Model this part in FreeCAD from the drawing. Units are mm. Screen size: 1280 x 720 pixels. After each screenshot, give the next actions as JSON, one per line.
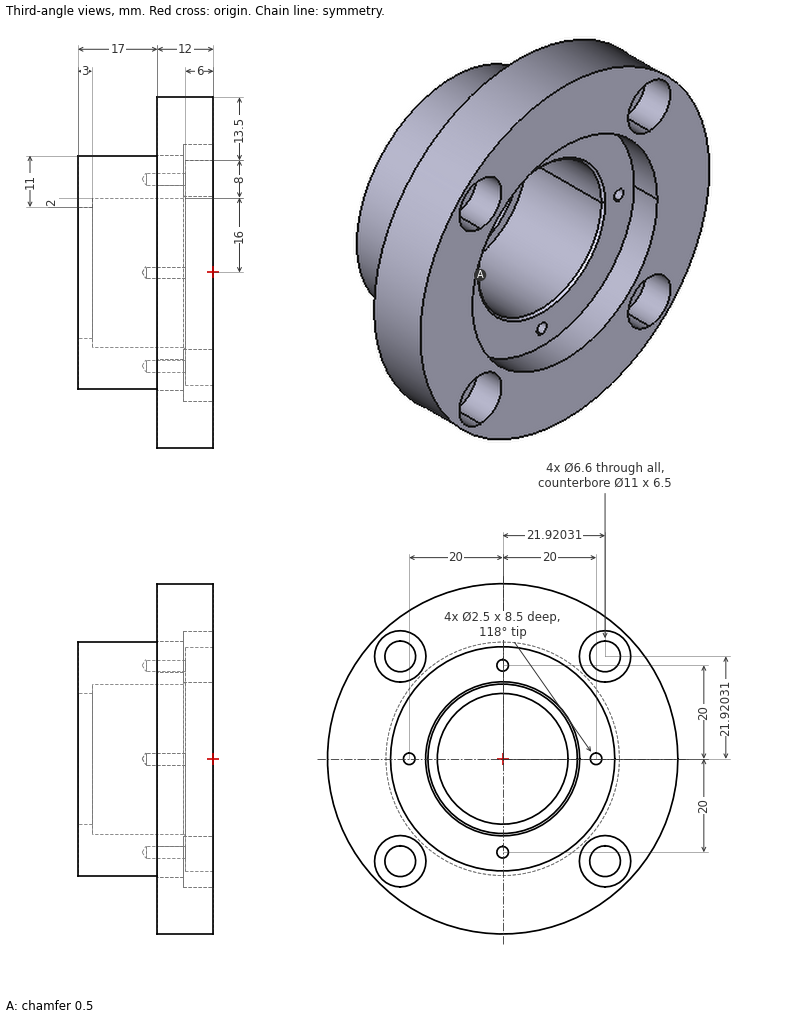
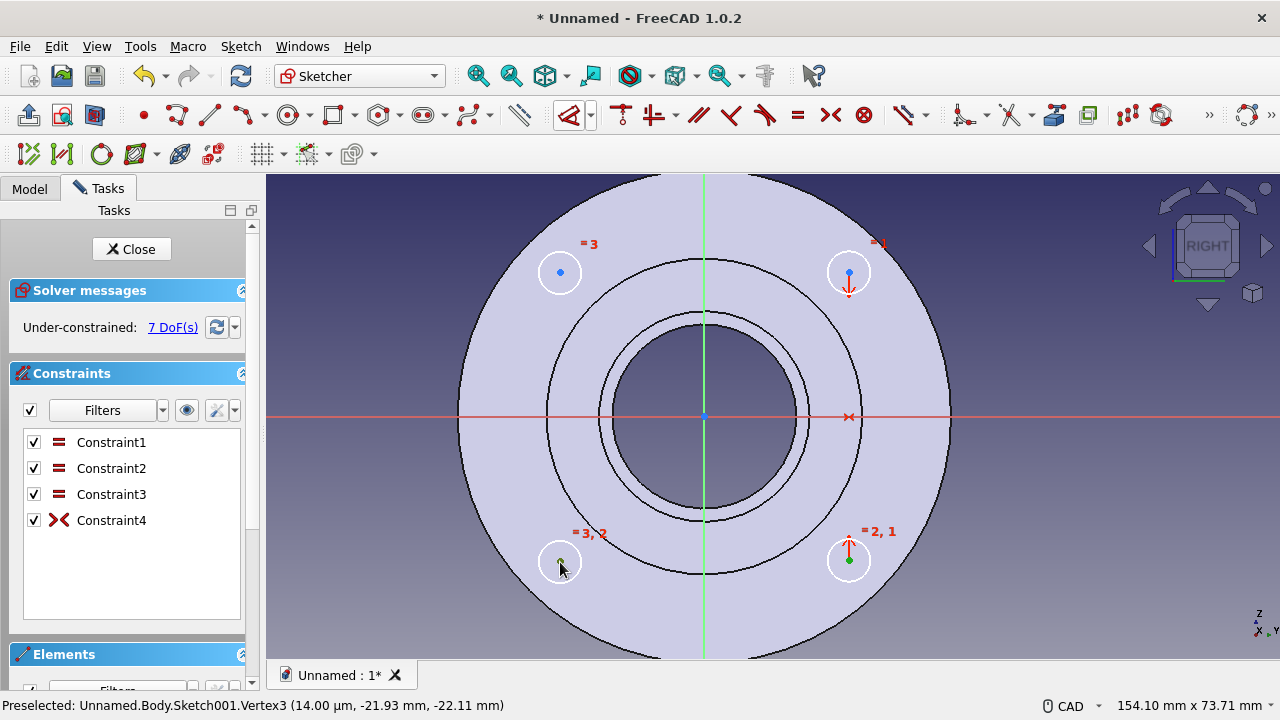
{"action": "left_click", "coordinate": [704, 600]}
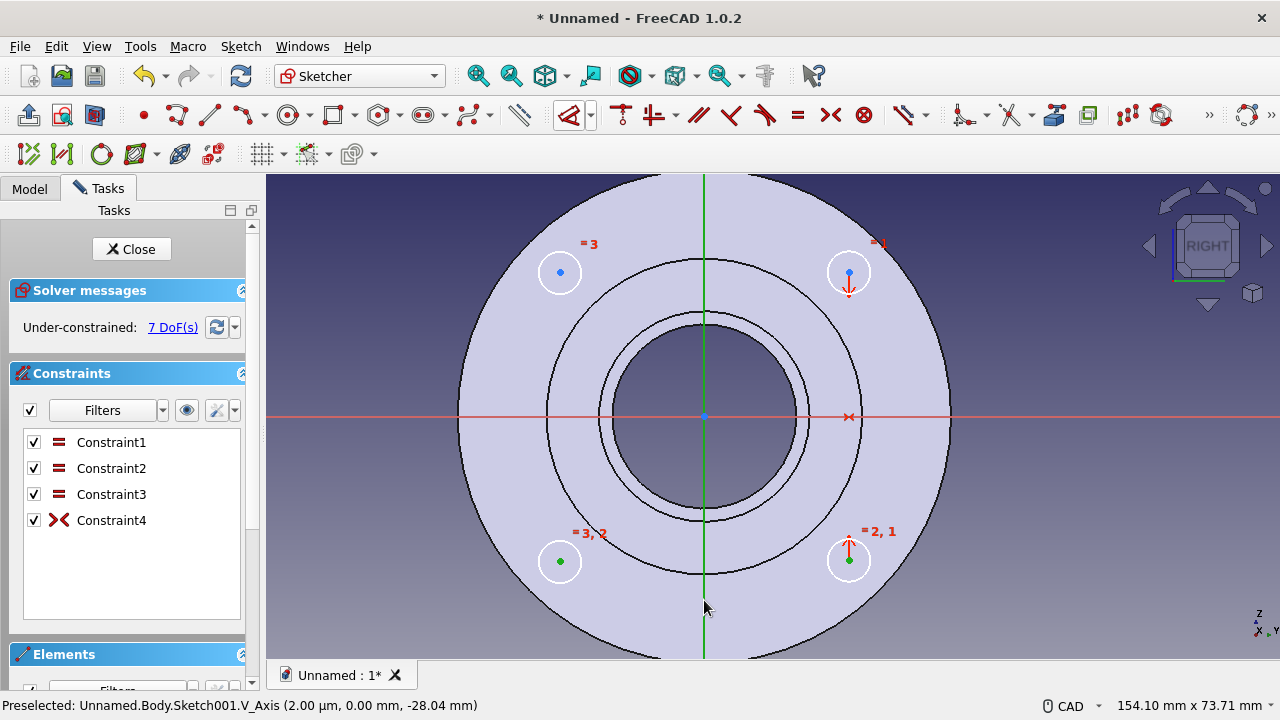
{"action": "key", "text": "s"}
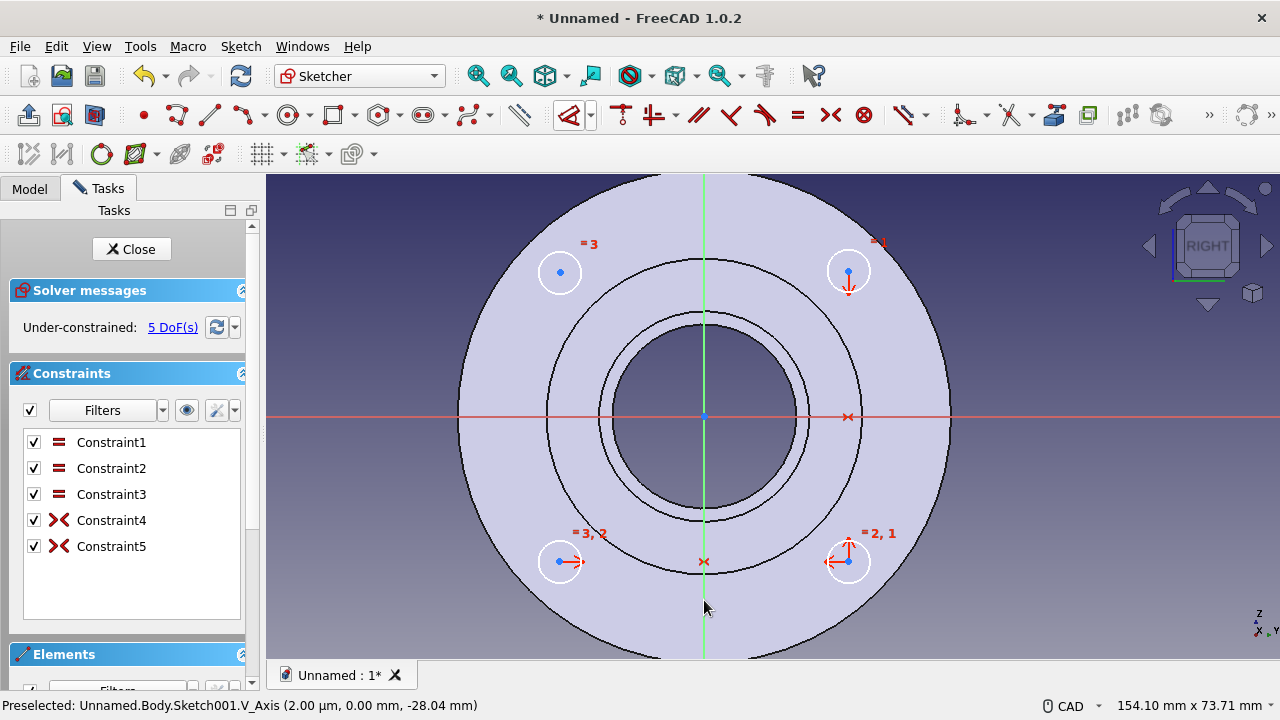
{"action": "left_click", "coordinate": [849, 271]}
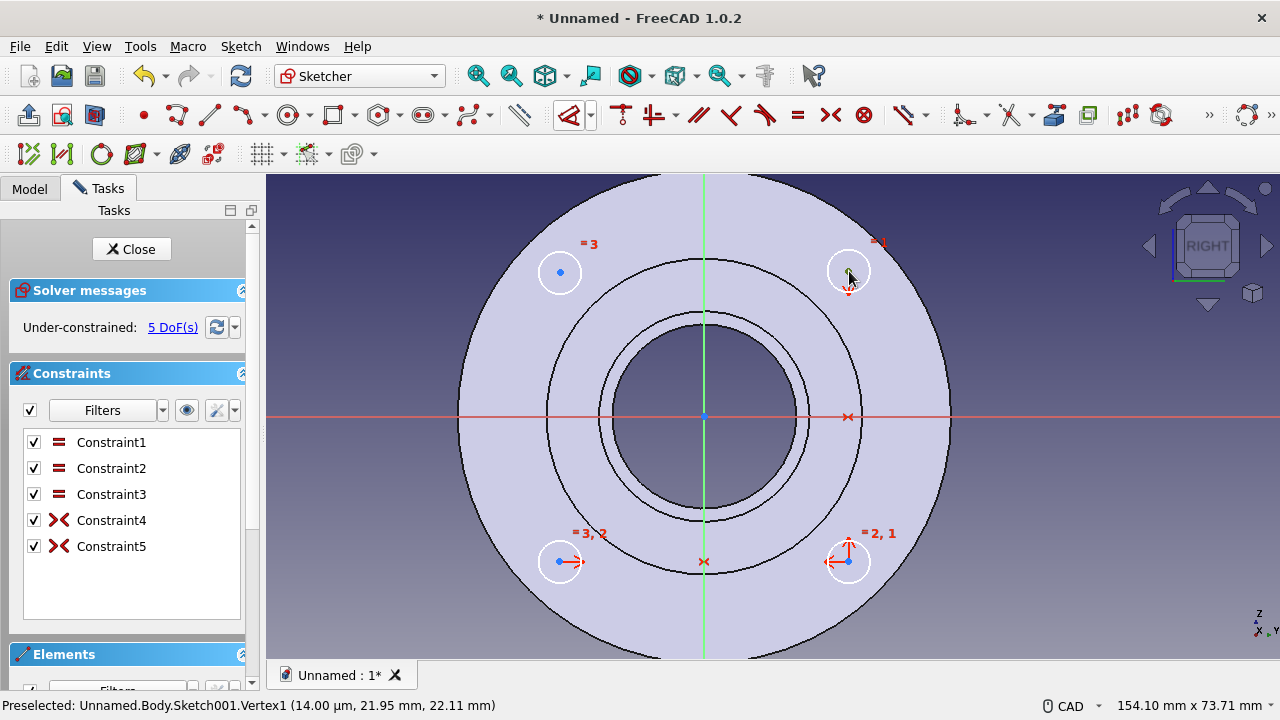
{"action": "left_click", "coordinate": [560, 273]}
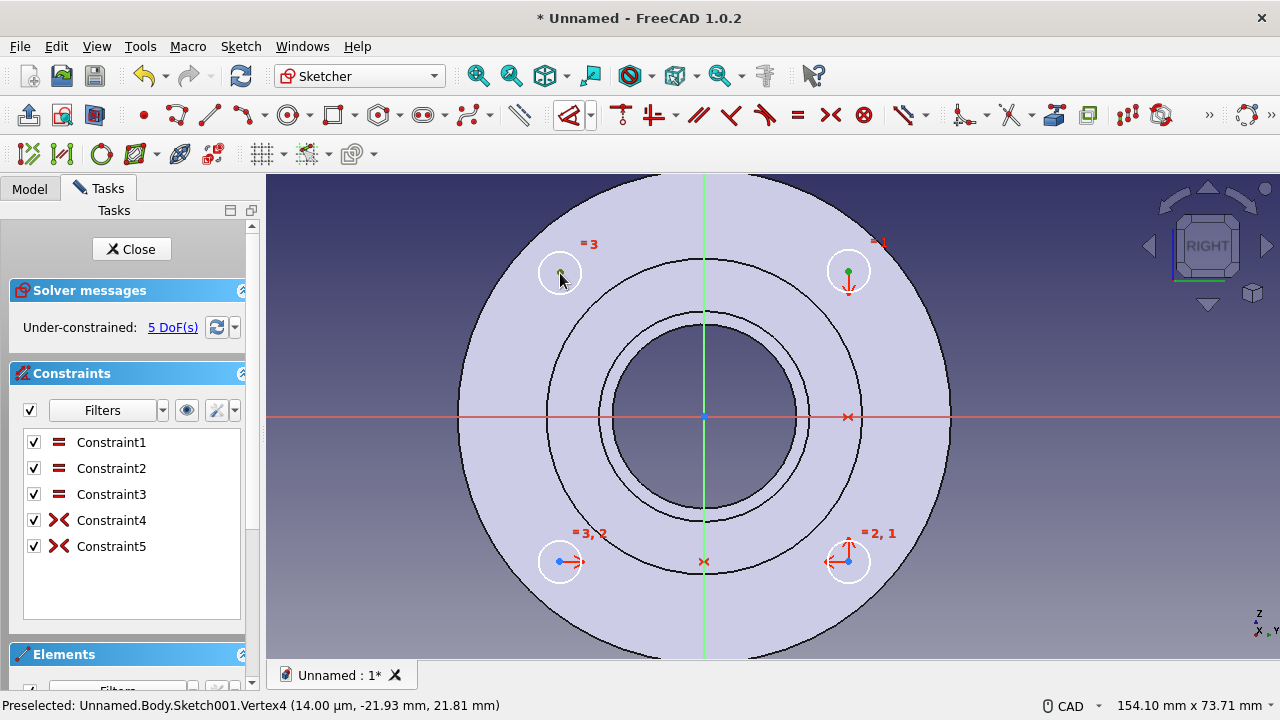
{"action": "left_click", "coordinate": [704, 600]}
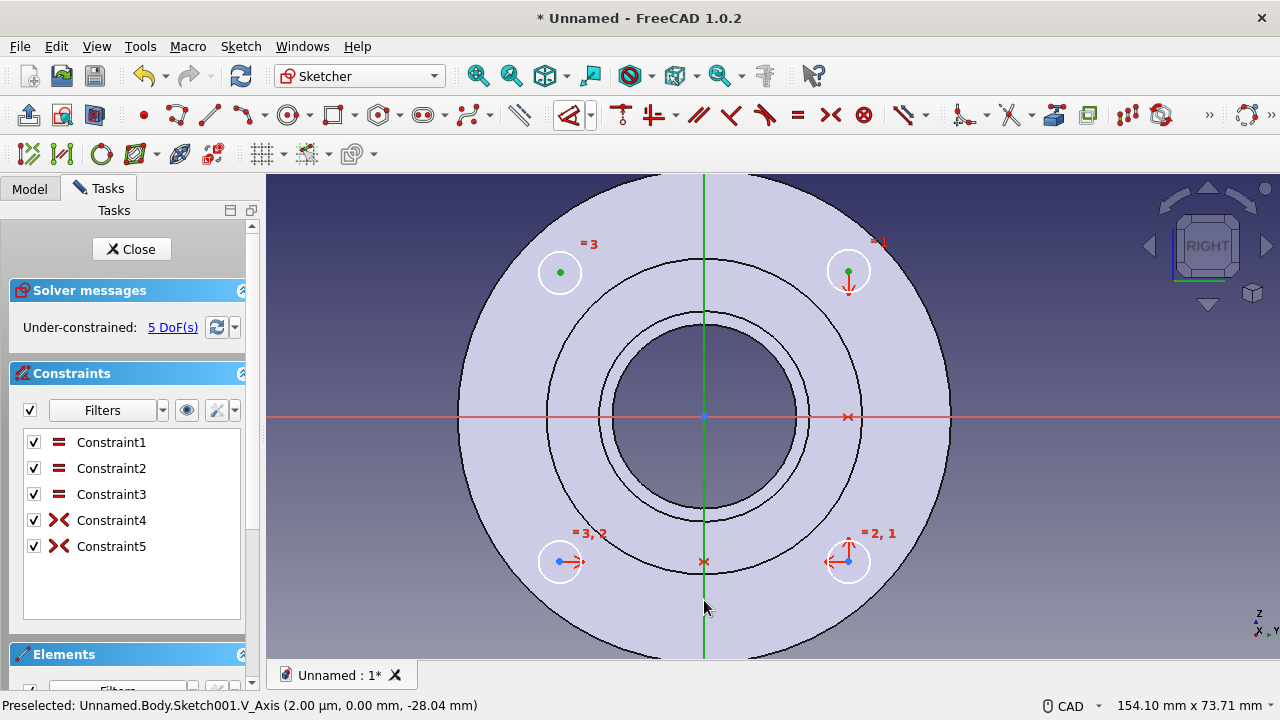
{"action": "key", "text": "s"}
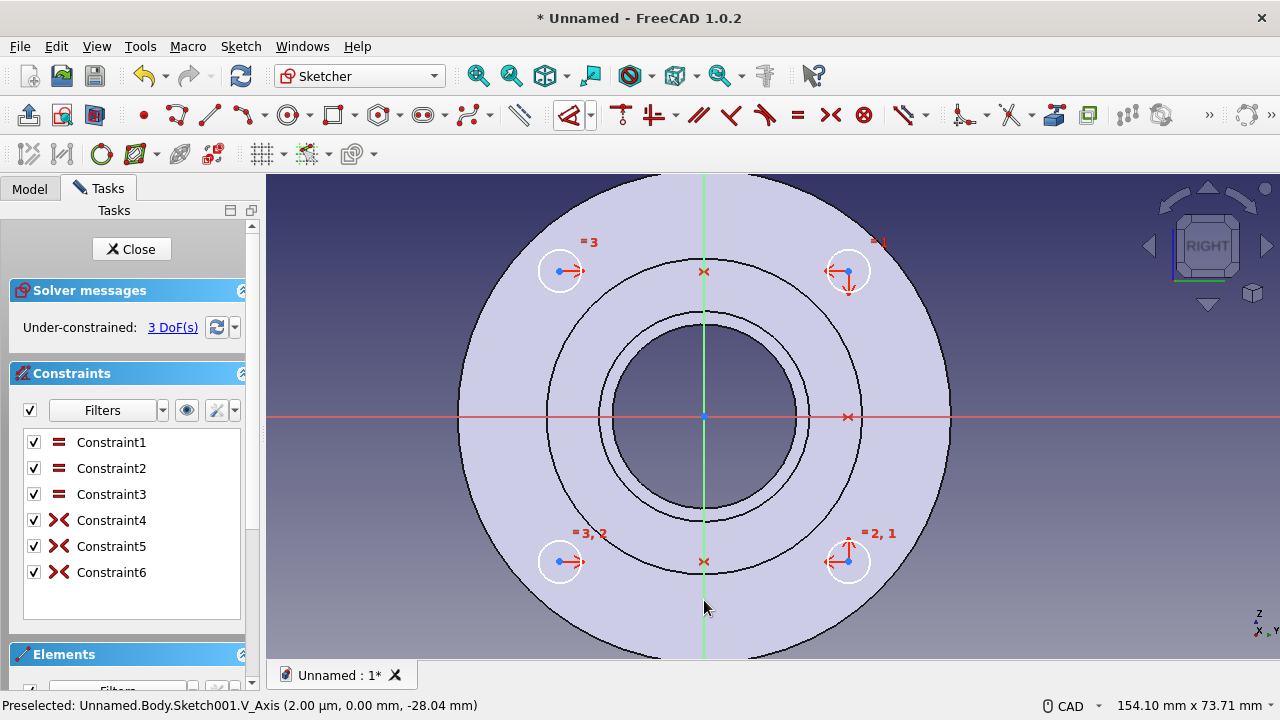
{"action": "left_click", "coordinate": [864, 256]}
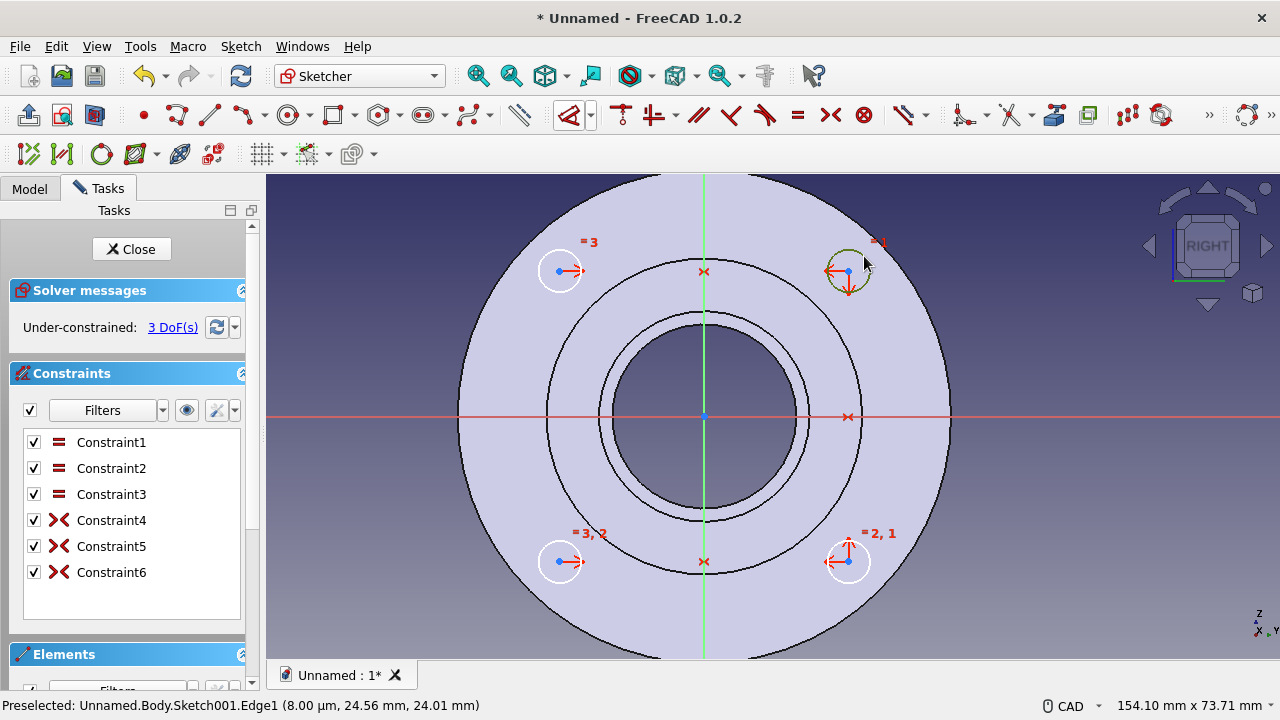
{"action": "key", "text": "k o"}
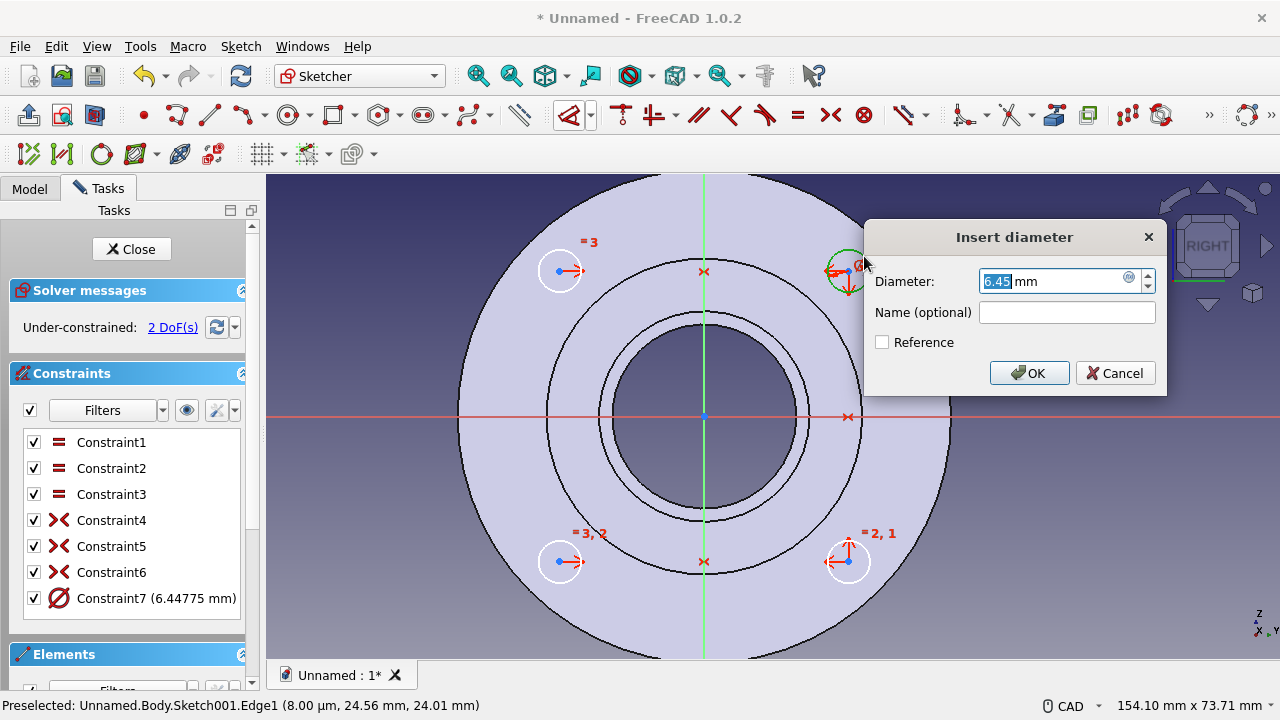
{"action": "type", "text": "6.6"}
{"action": "key", "text": "Return"}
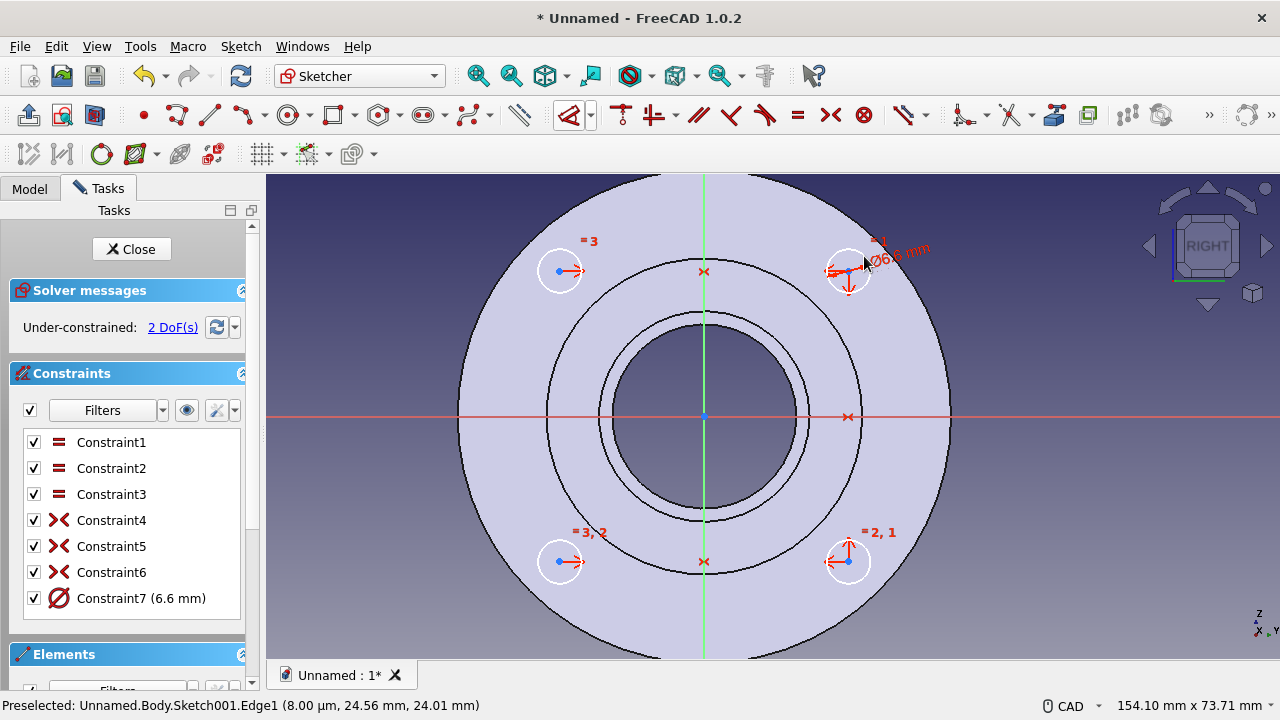
{"action": "left_click", "coordinate": [849, 271]}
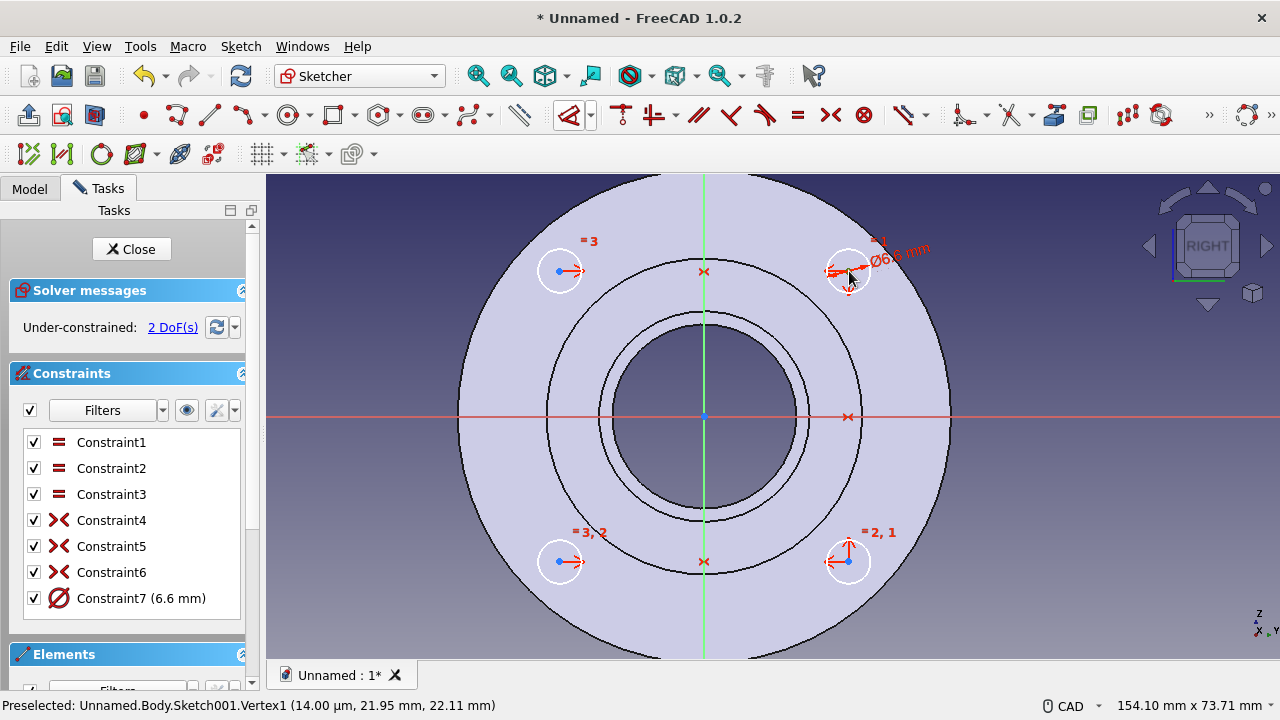
{"action": "key", "text": "l"}